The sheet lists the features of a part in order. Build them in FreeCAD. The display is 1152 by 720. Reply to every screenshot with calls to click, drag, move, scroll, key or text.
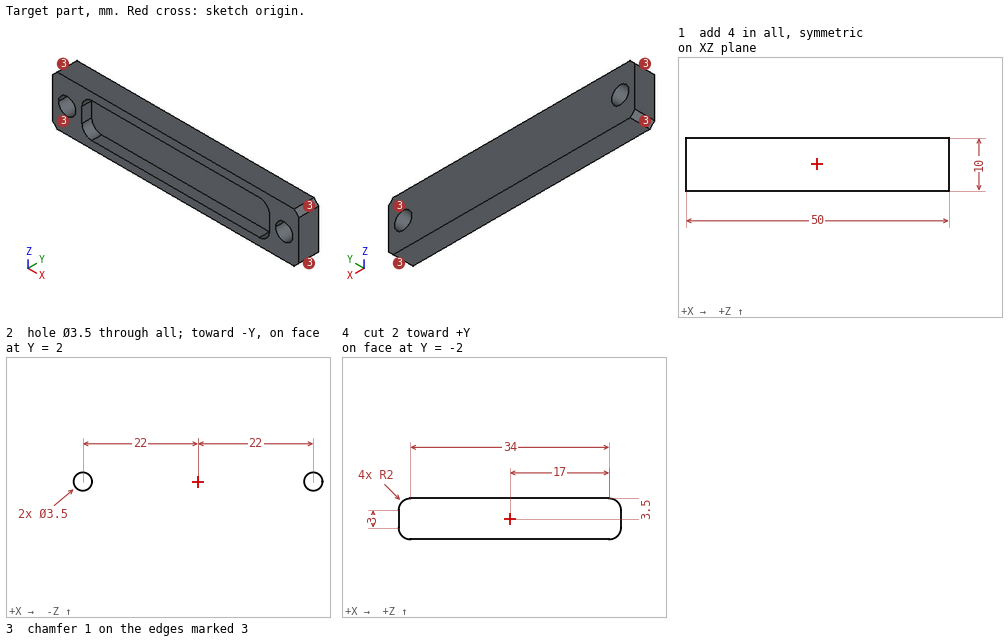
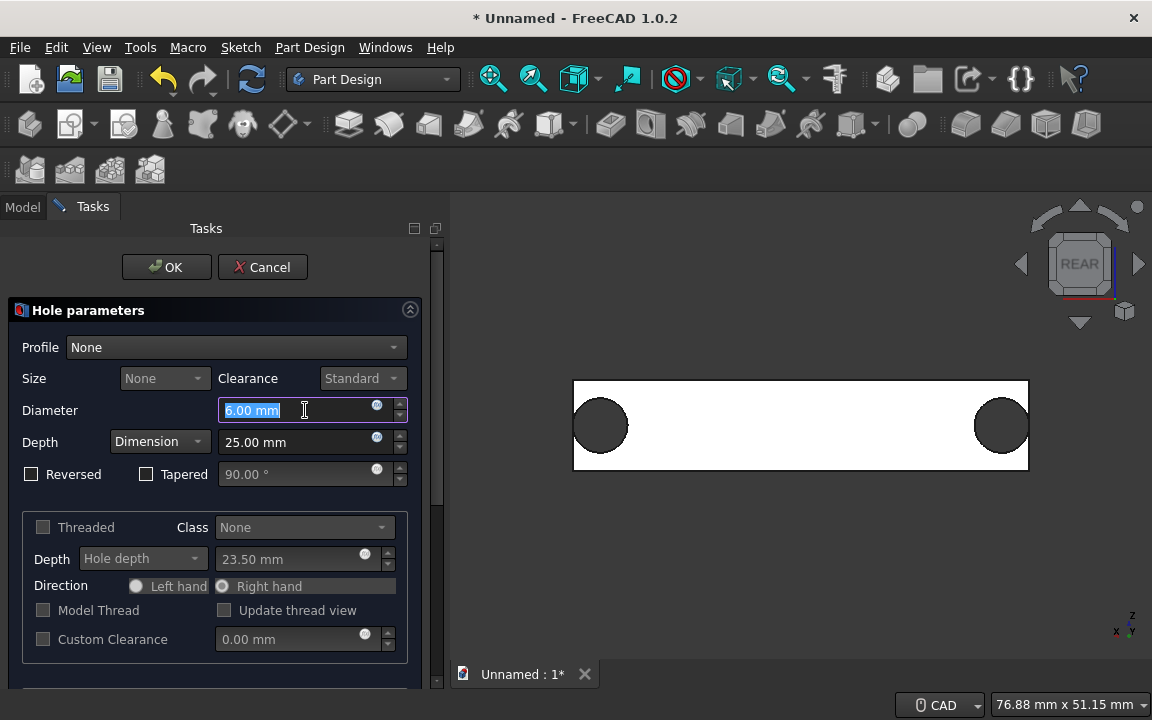
text(3.5)
key(Tab)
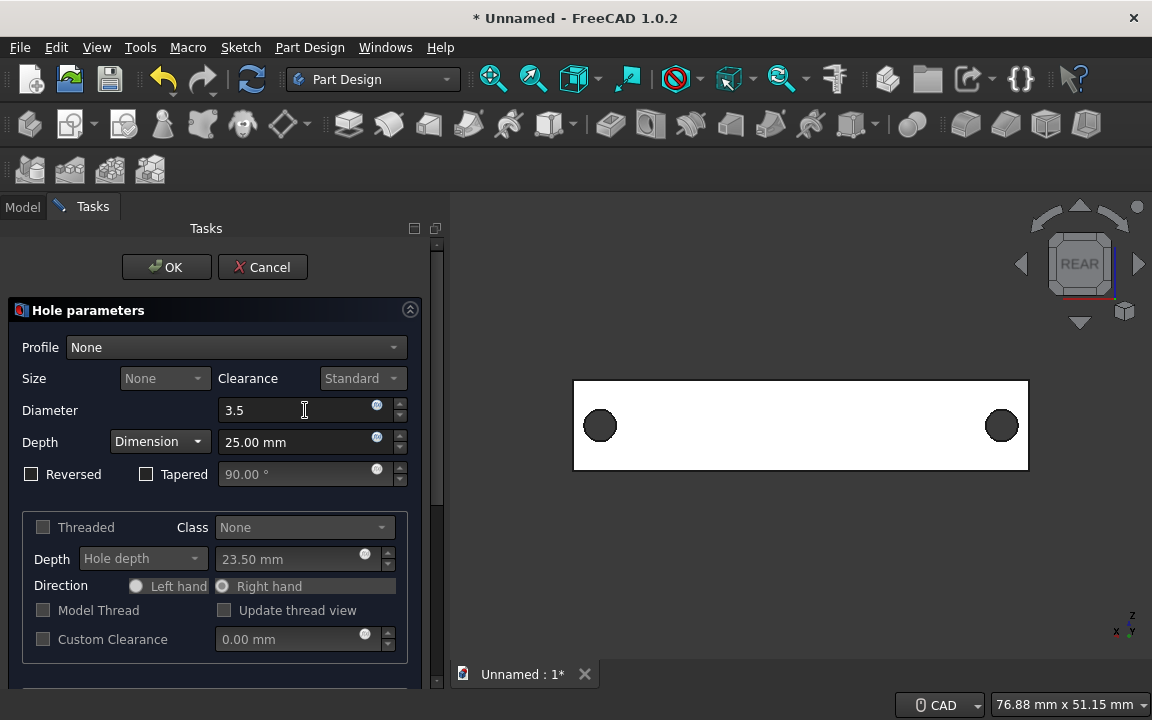
click(161, 442)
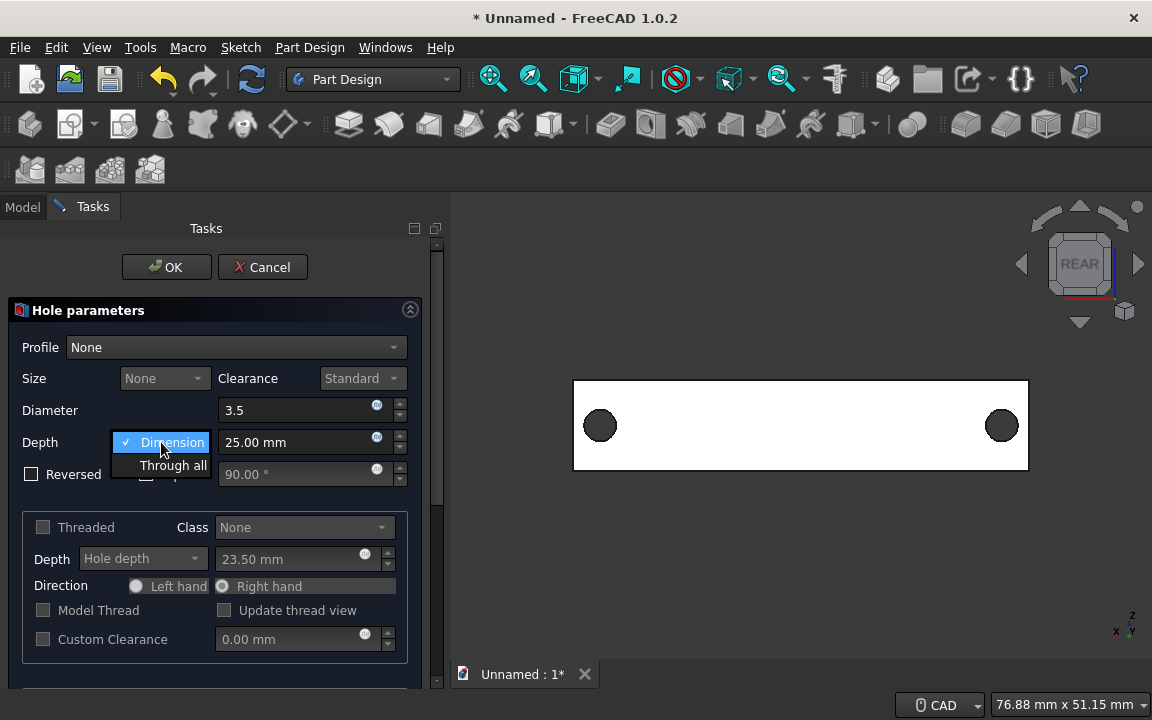
click(160, 466)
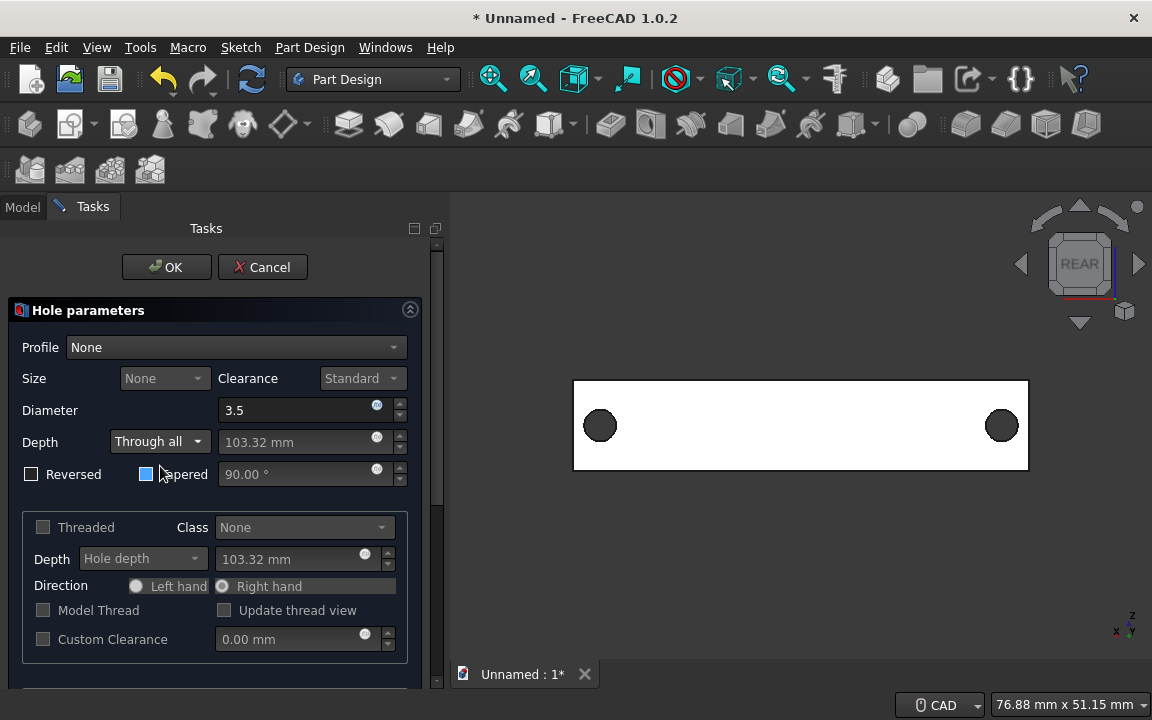
click(167, 267)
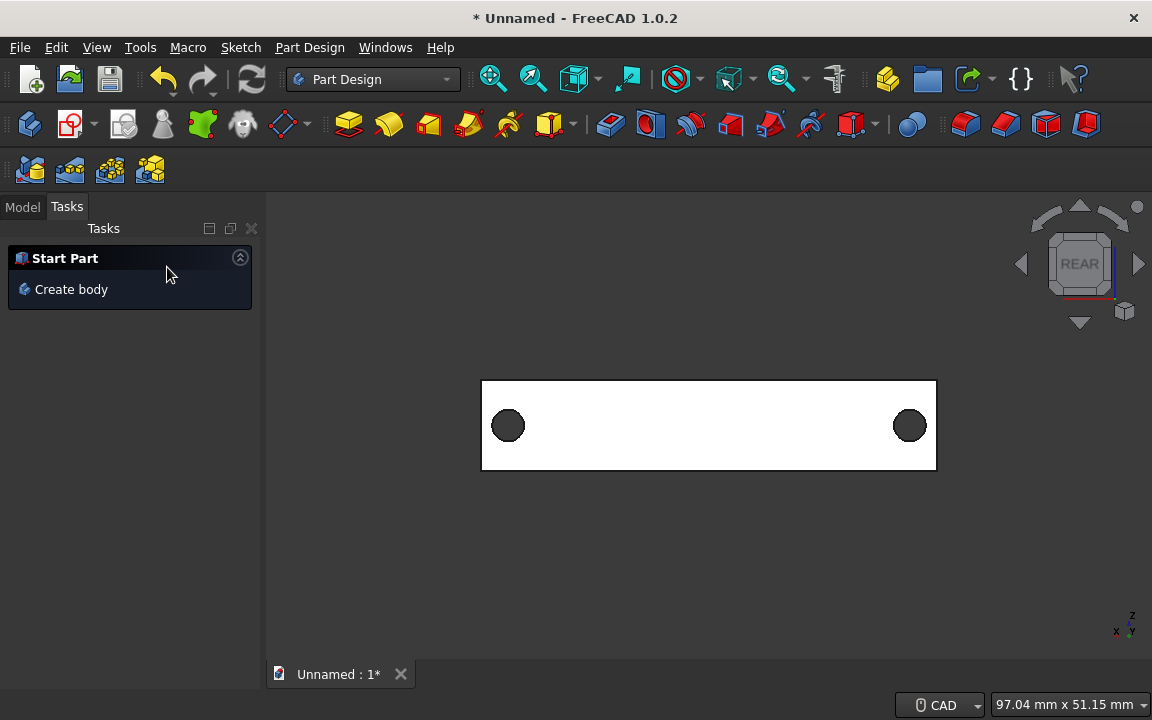
key(0)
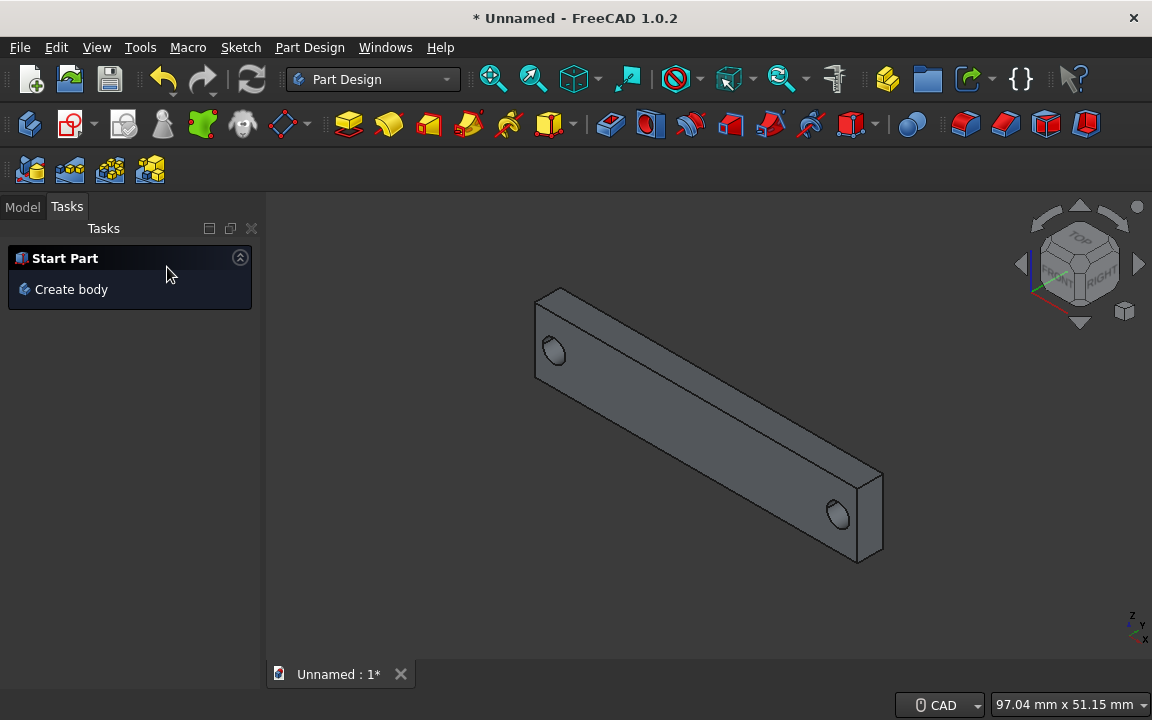
click(870, 480)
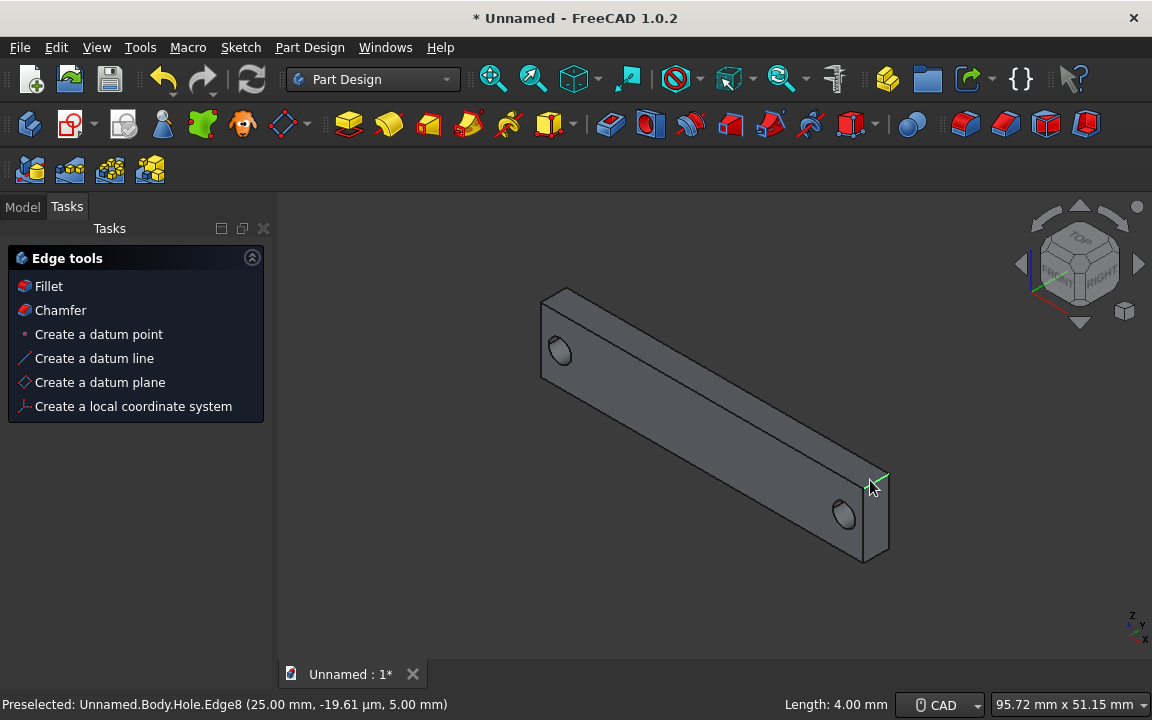
key(2)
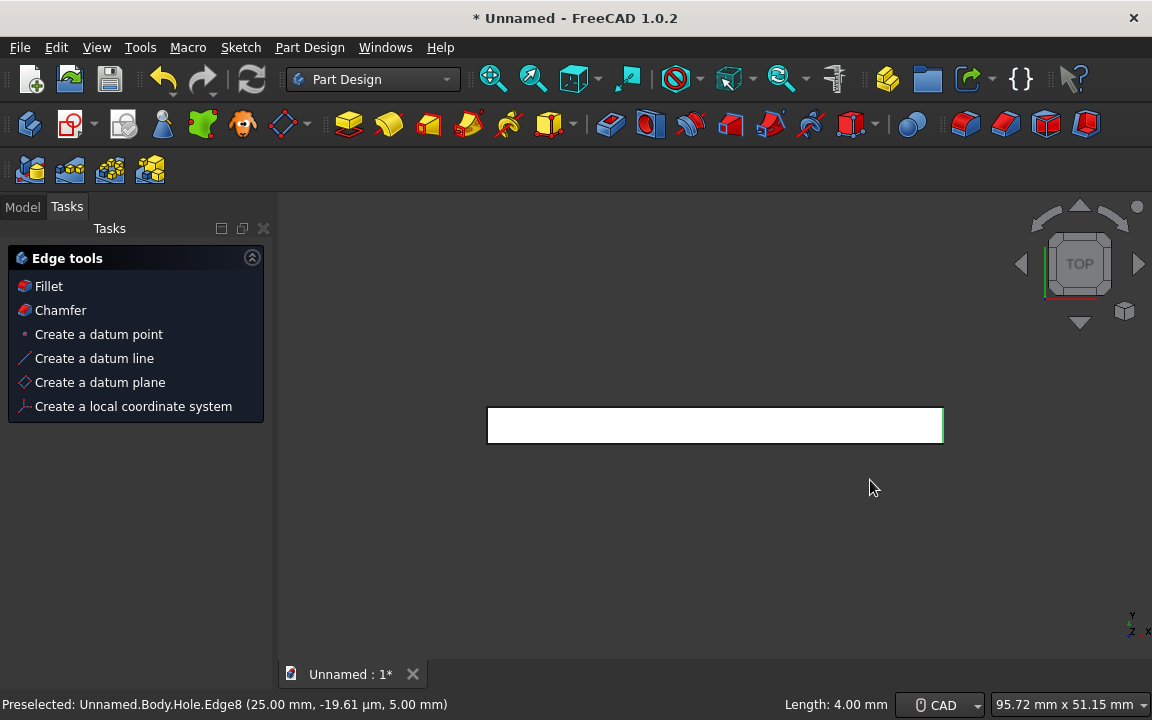
click(487, 424, ctrl)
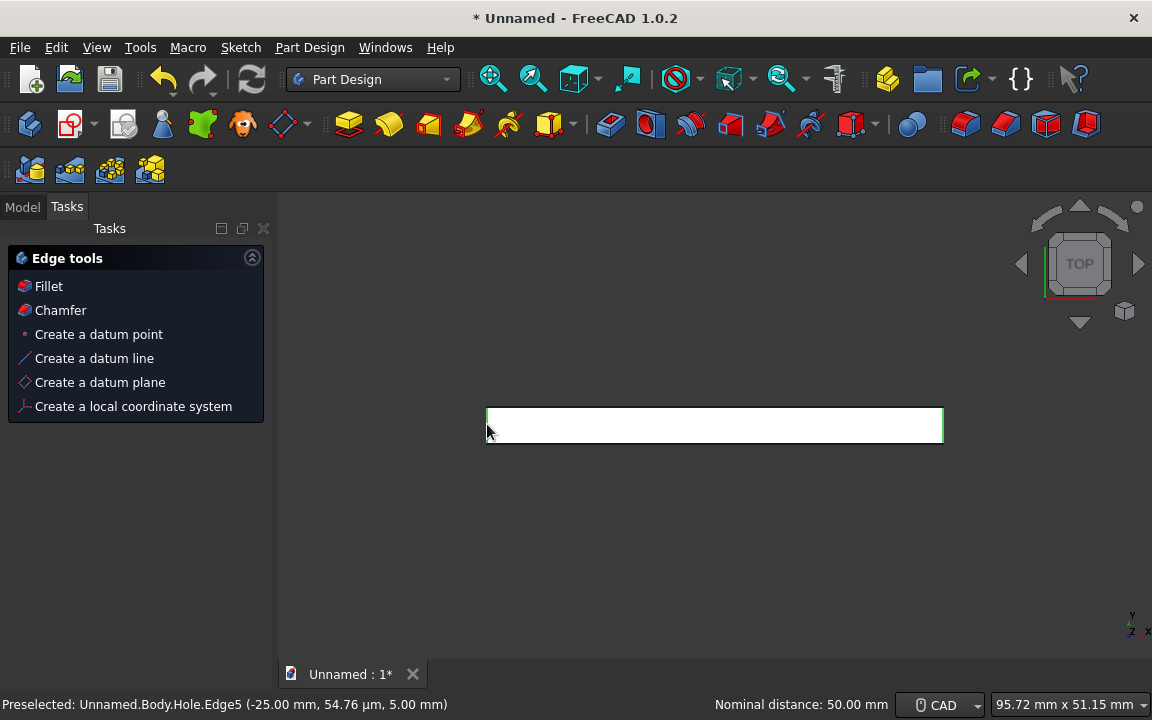
key(1)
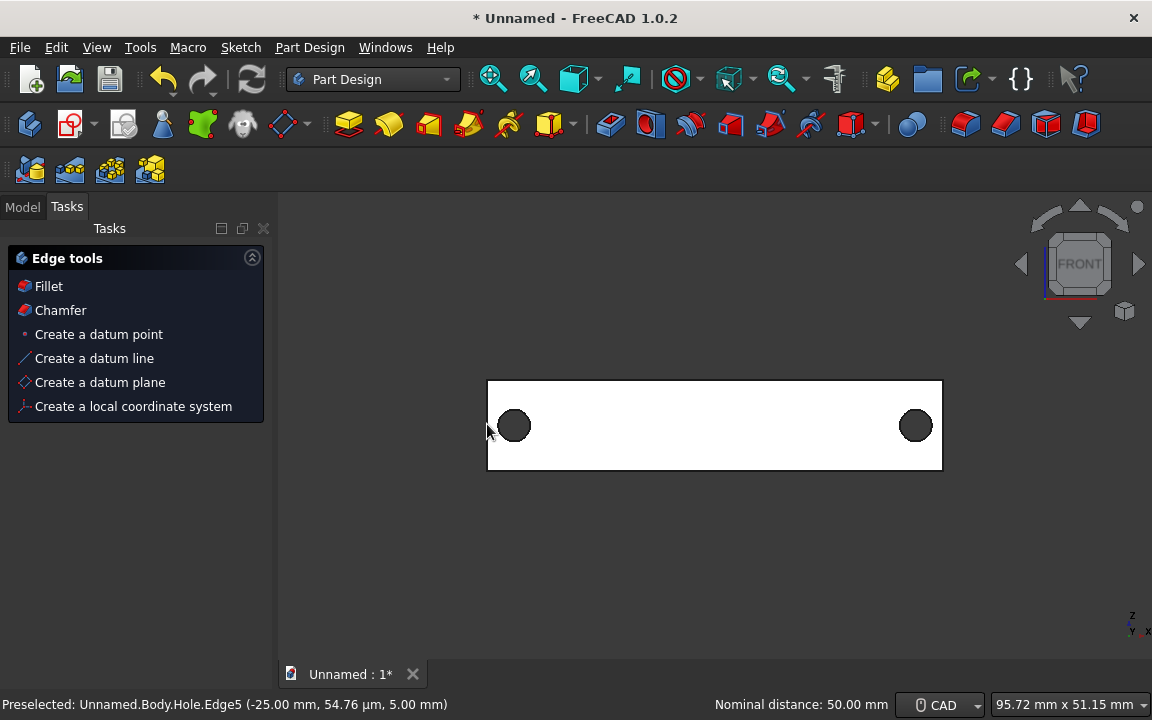
key(3)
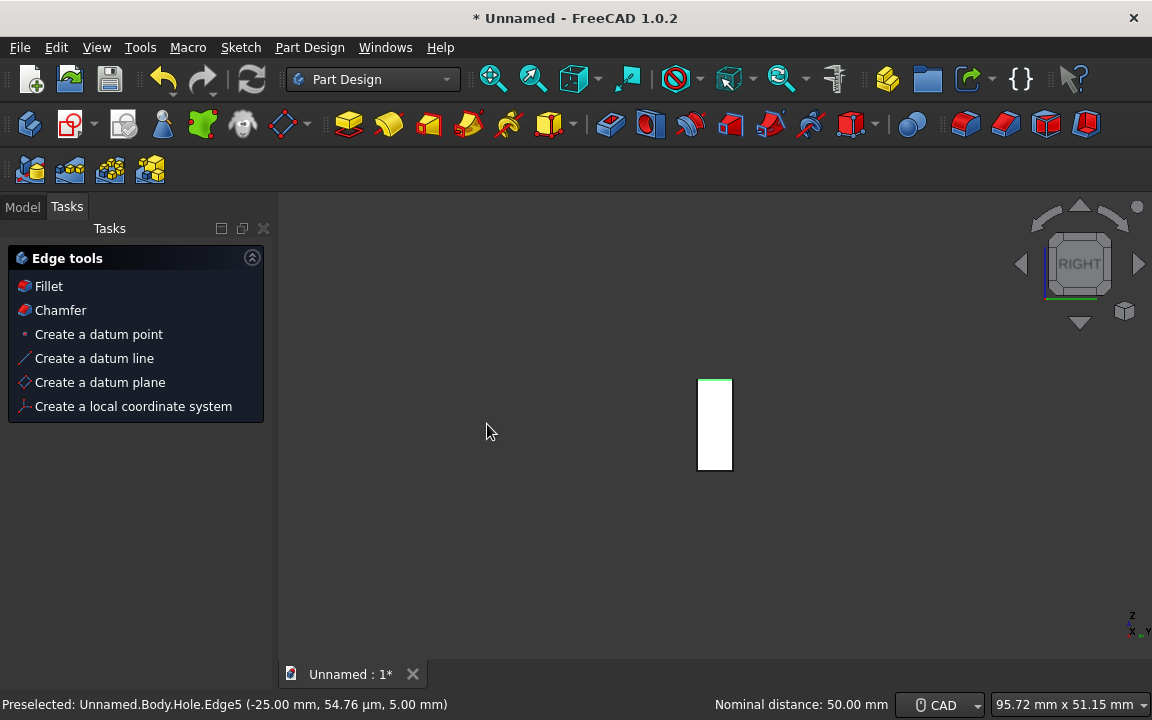
click(494, 80)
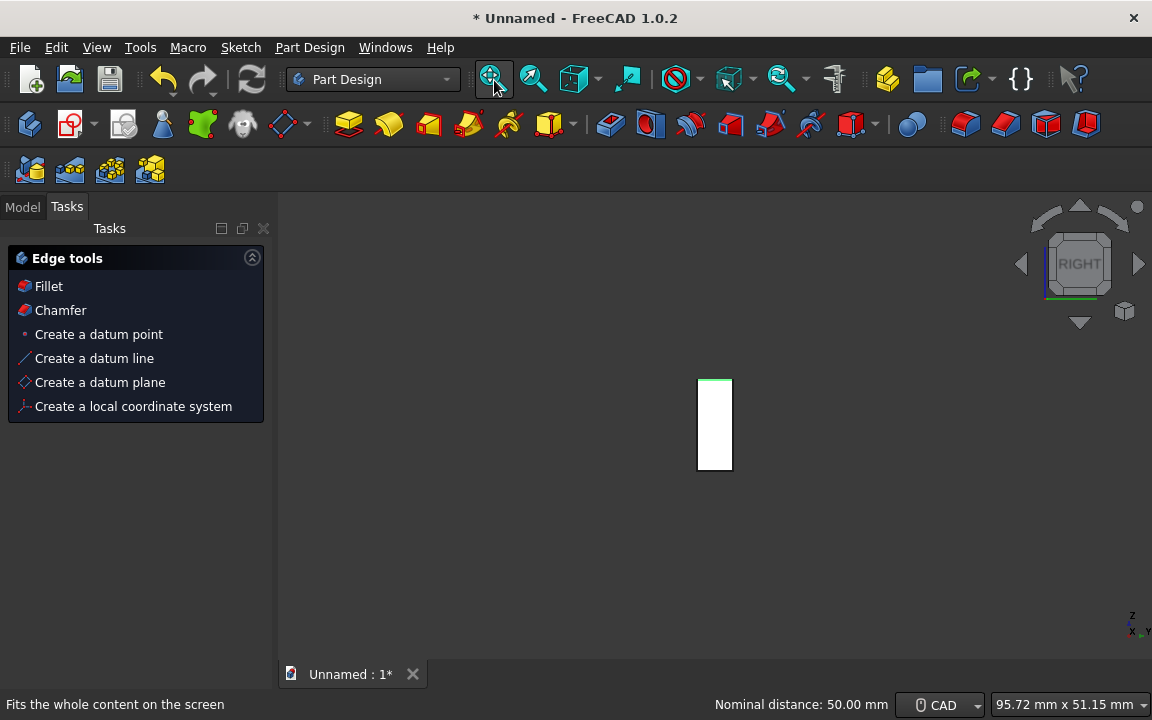
click(715, 470, ctrl)